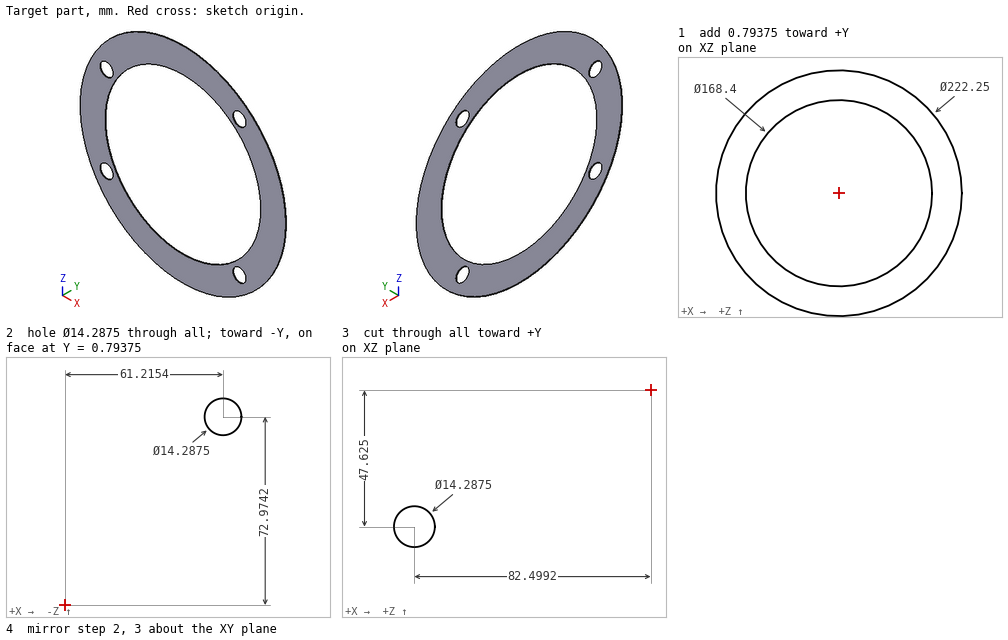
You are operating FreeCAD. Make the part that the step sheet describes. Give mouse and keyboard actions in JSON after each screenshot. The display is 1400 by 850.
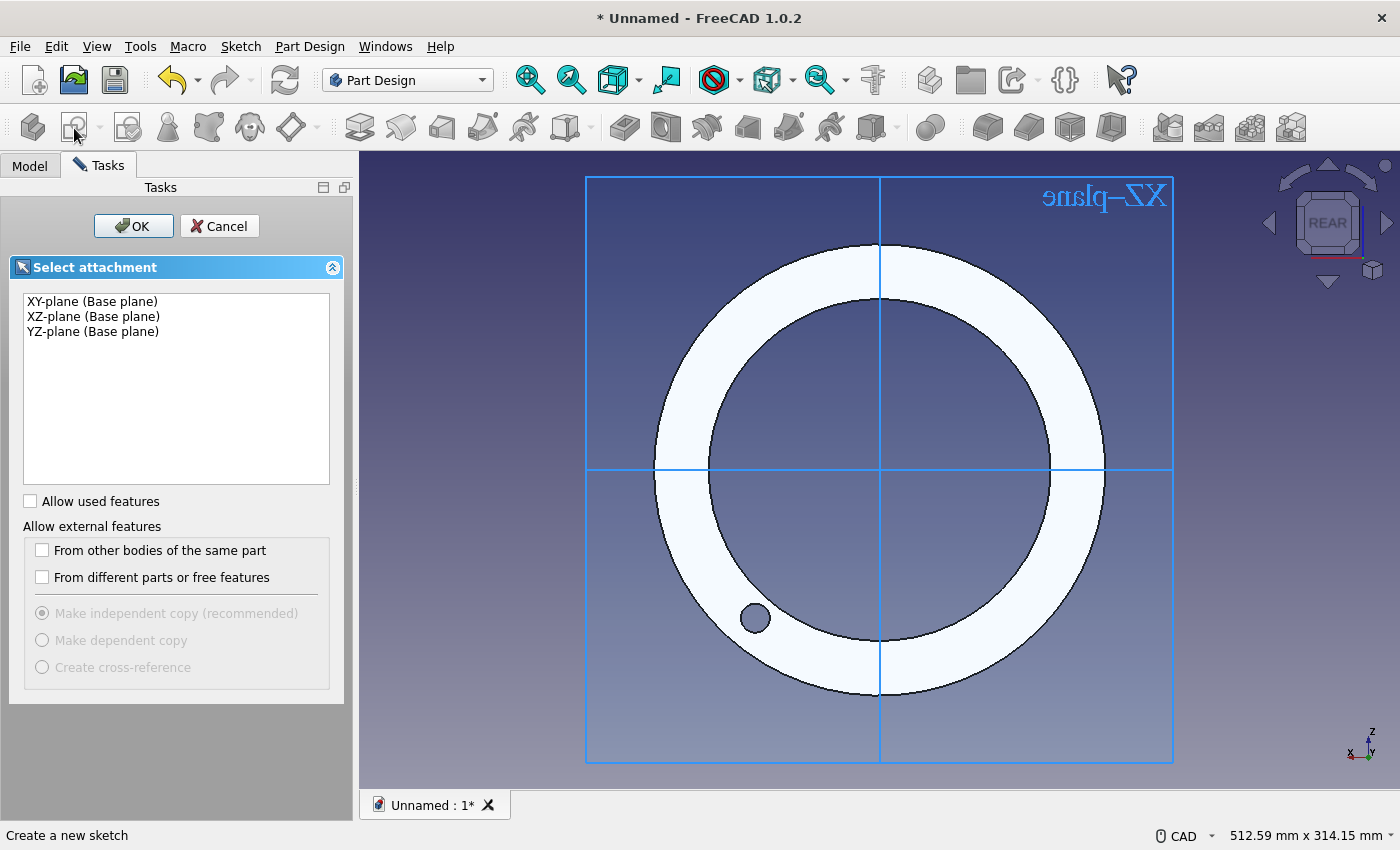
{"action": "left_click", "coordinate": [84, 316]}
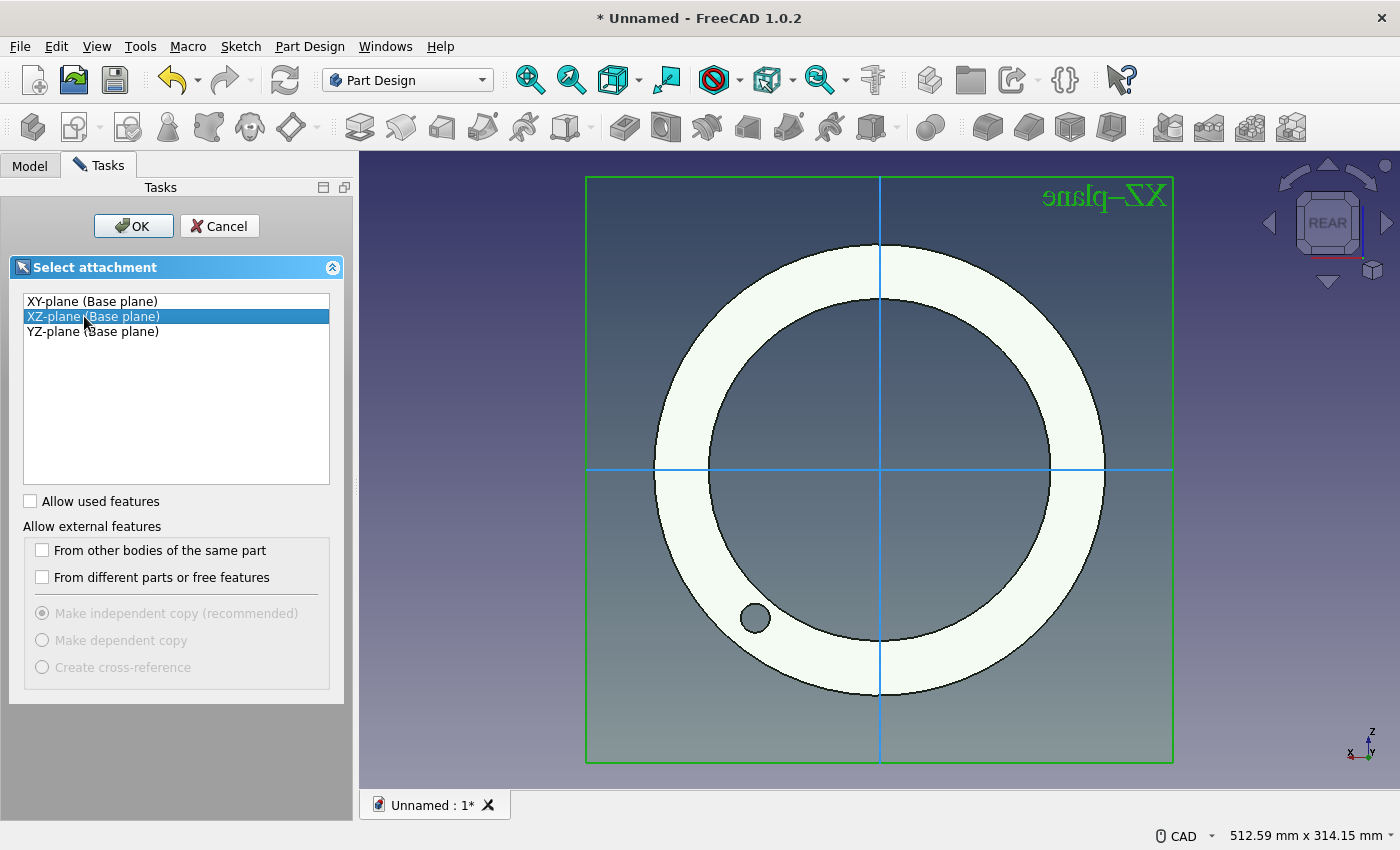
{"action": "left_click", "coordinate": [134, 226]}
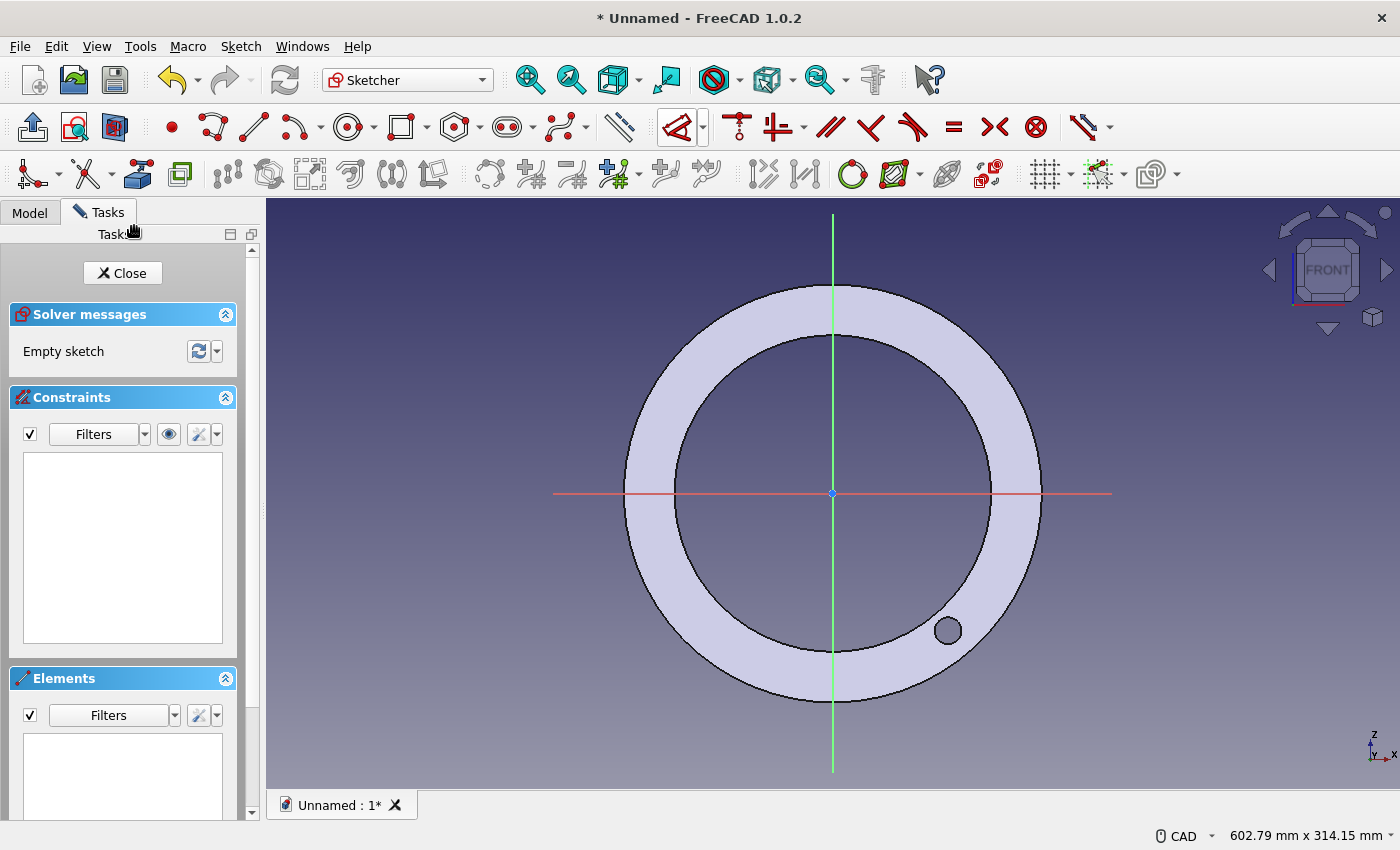
{"action": "scroll", "coordinate": [671, 590], "scroll_direction": "up", "scroll_amount": 13}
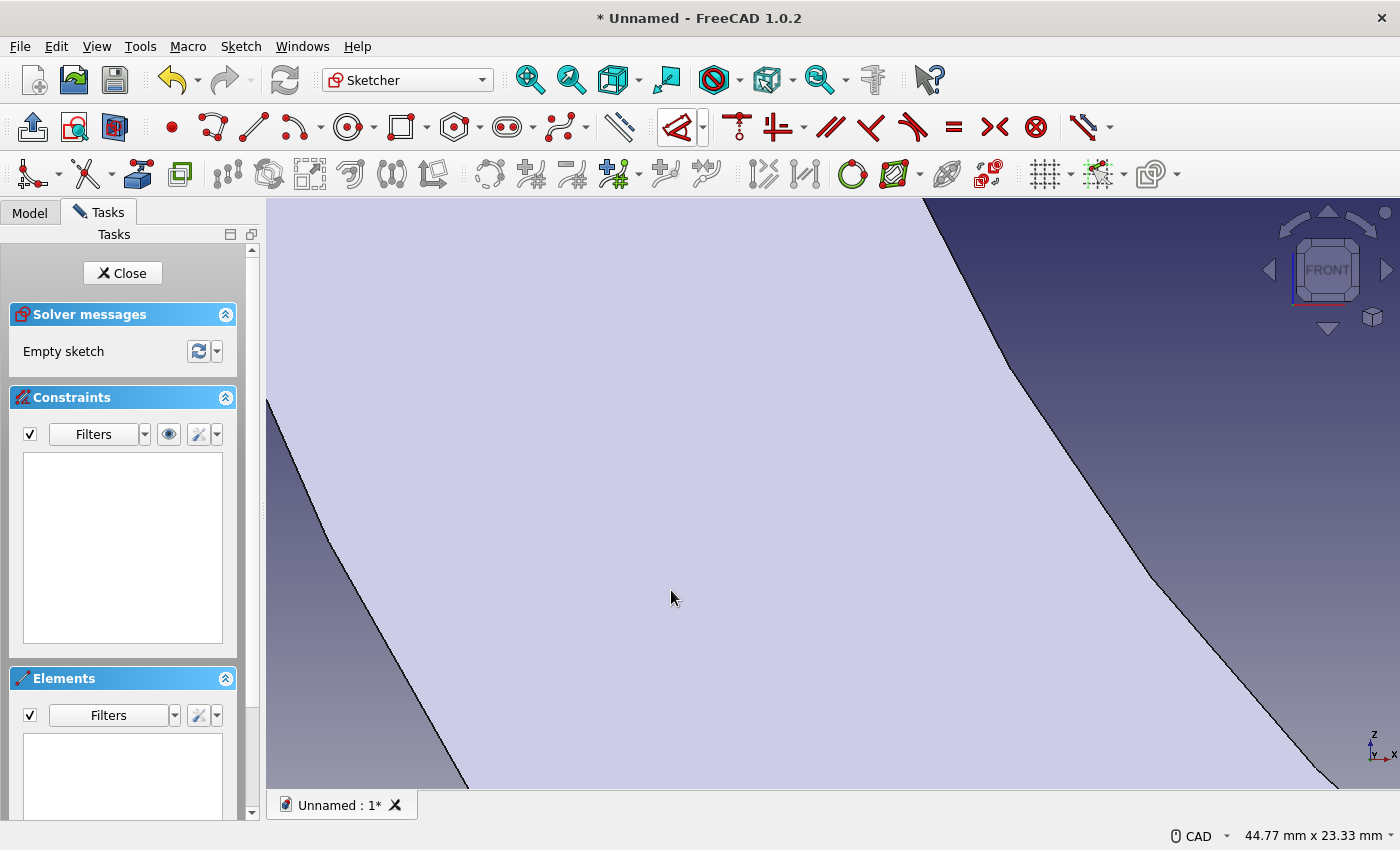
{"action": "left_click", "coordinate": [348, 128]}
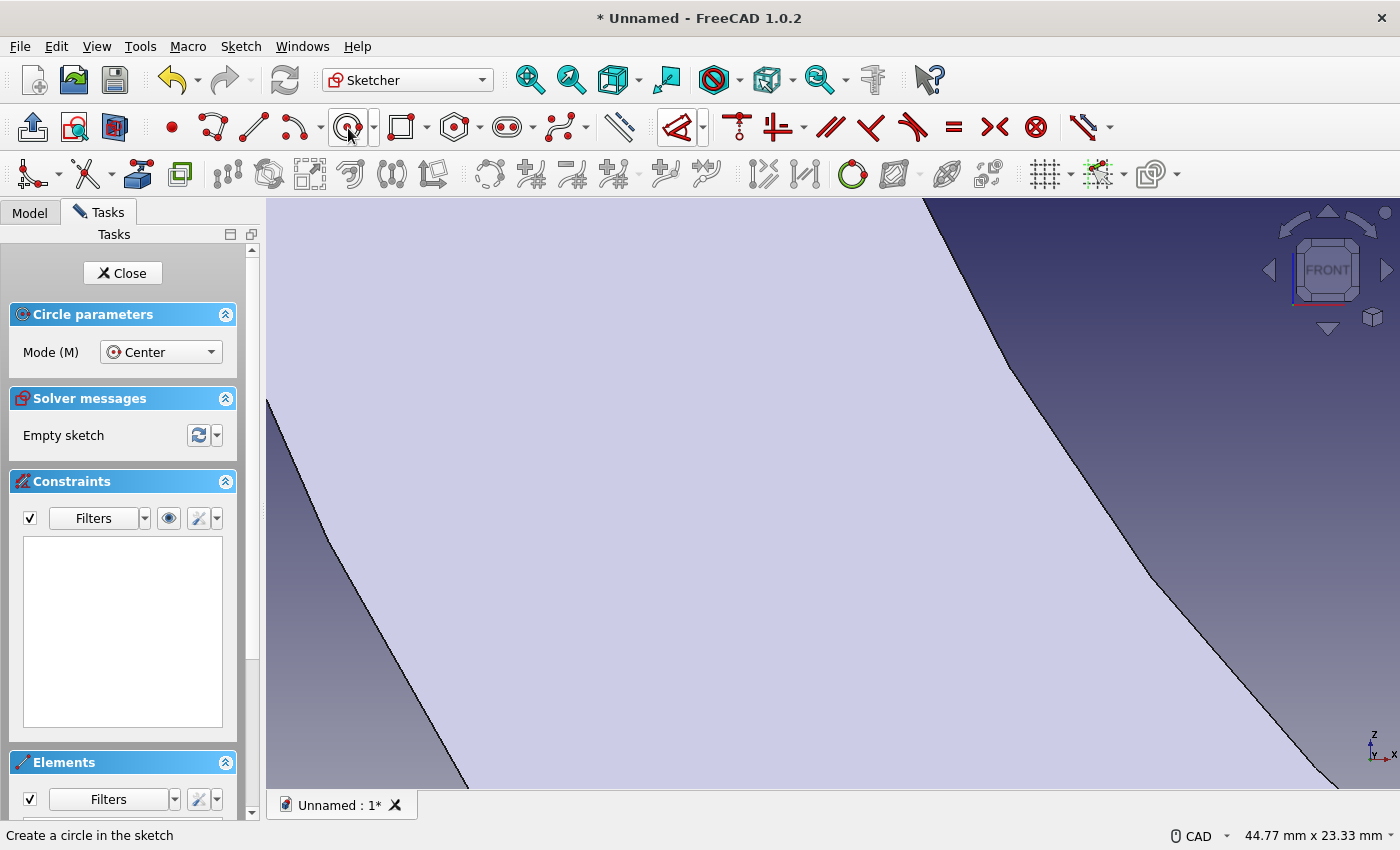
{"action": "left_click", "coordinate": [756, 489]}
{"action": "left_click", "coordinate": [884, 361]}
{"action": "key", "text": "Escape"}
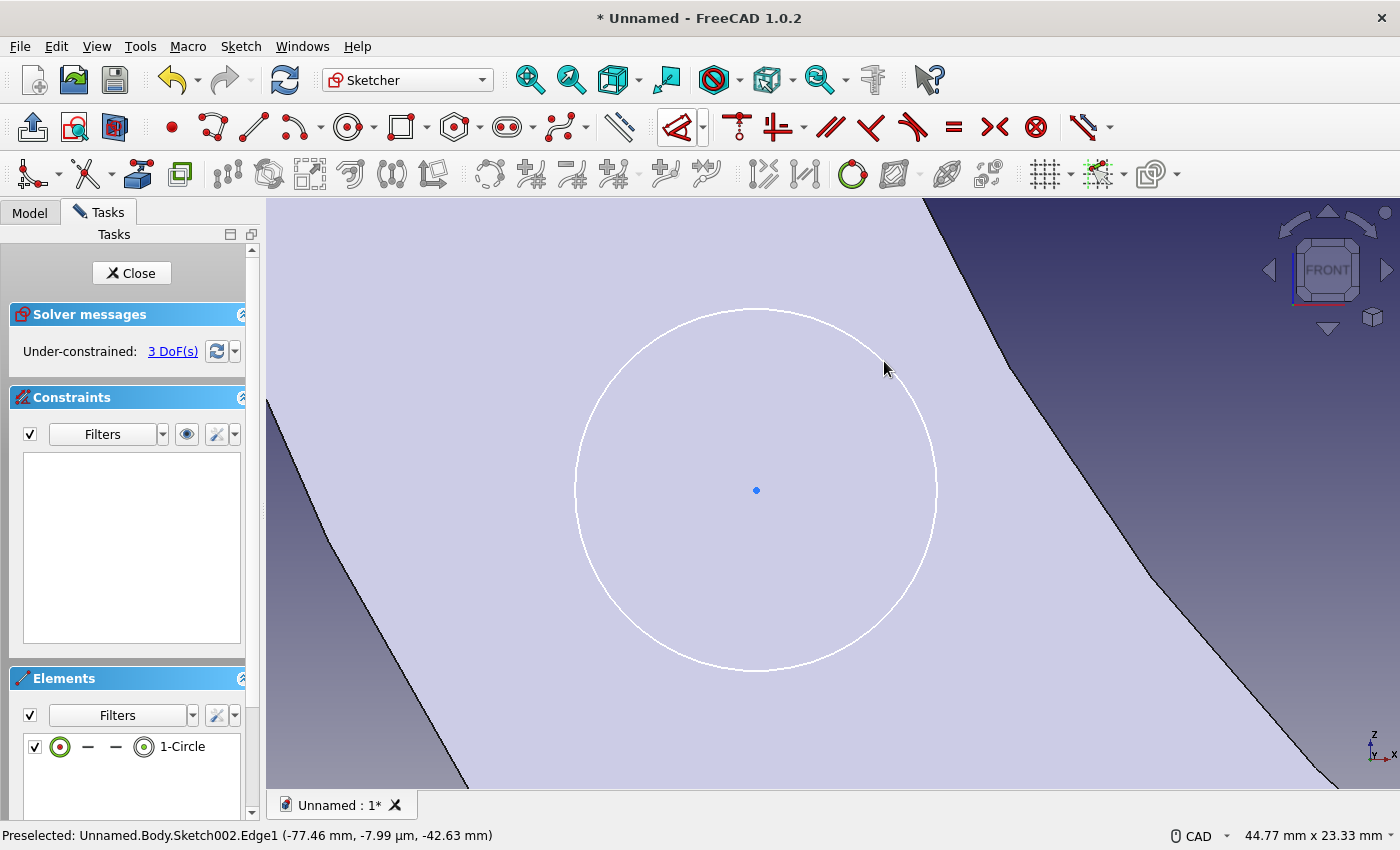
{"action": "left_click", "coordinate": [884, 362]}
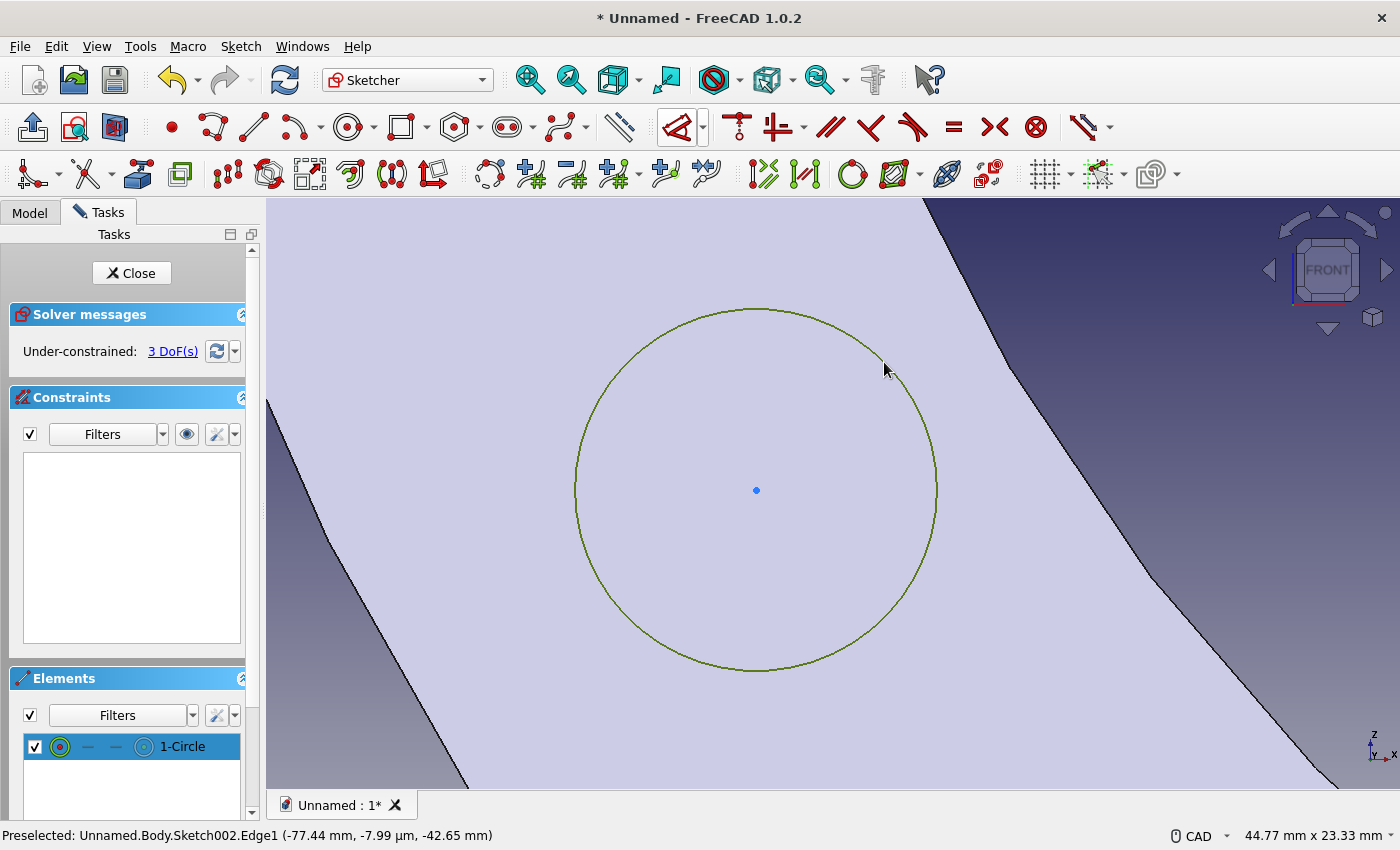
{"action": "key", "text": "k o"}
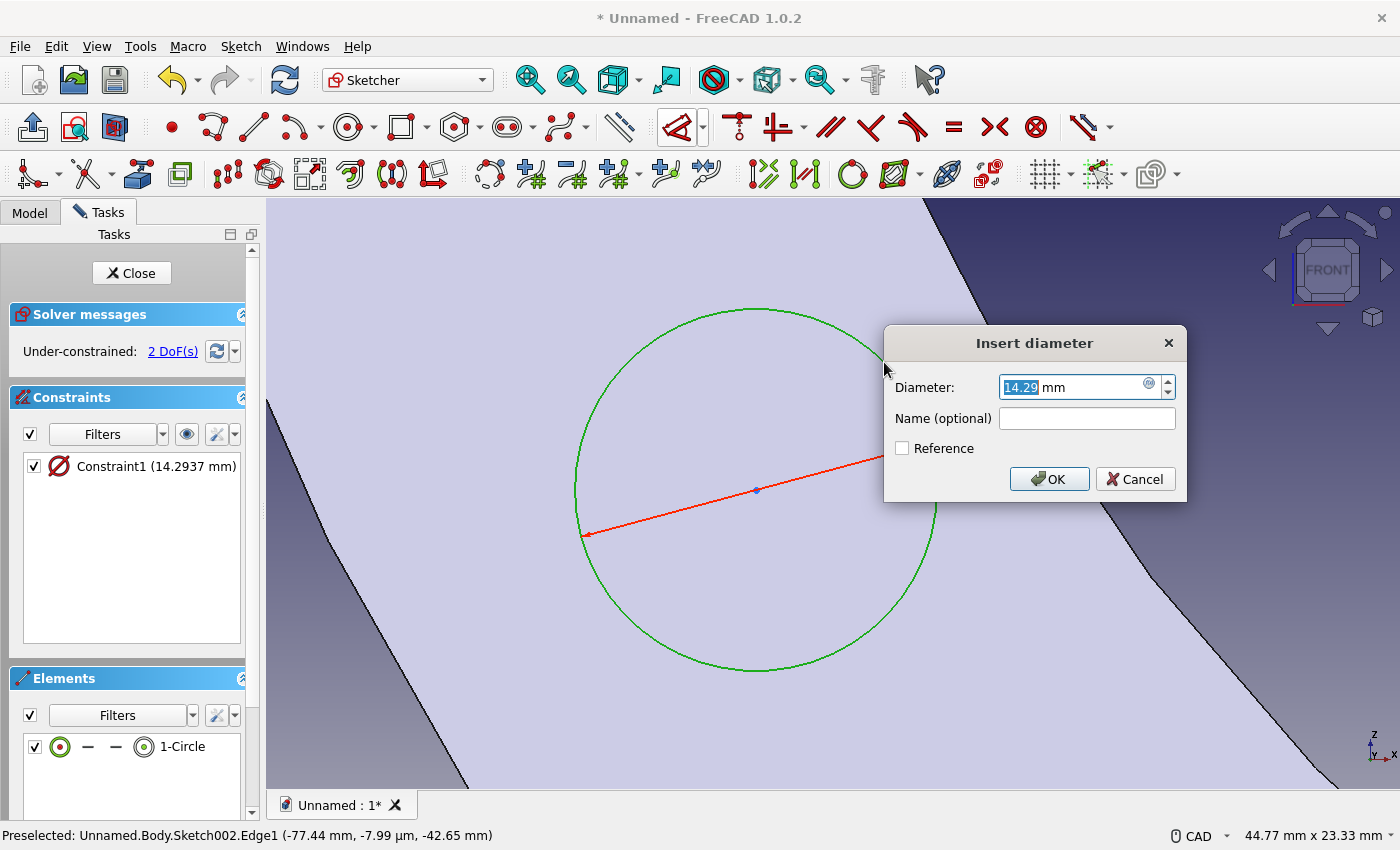
{"action": "type", "text": "14.2875"}
{"action": "key", "text": "Return"}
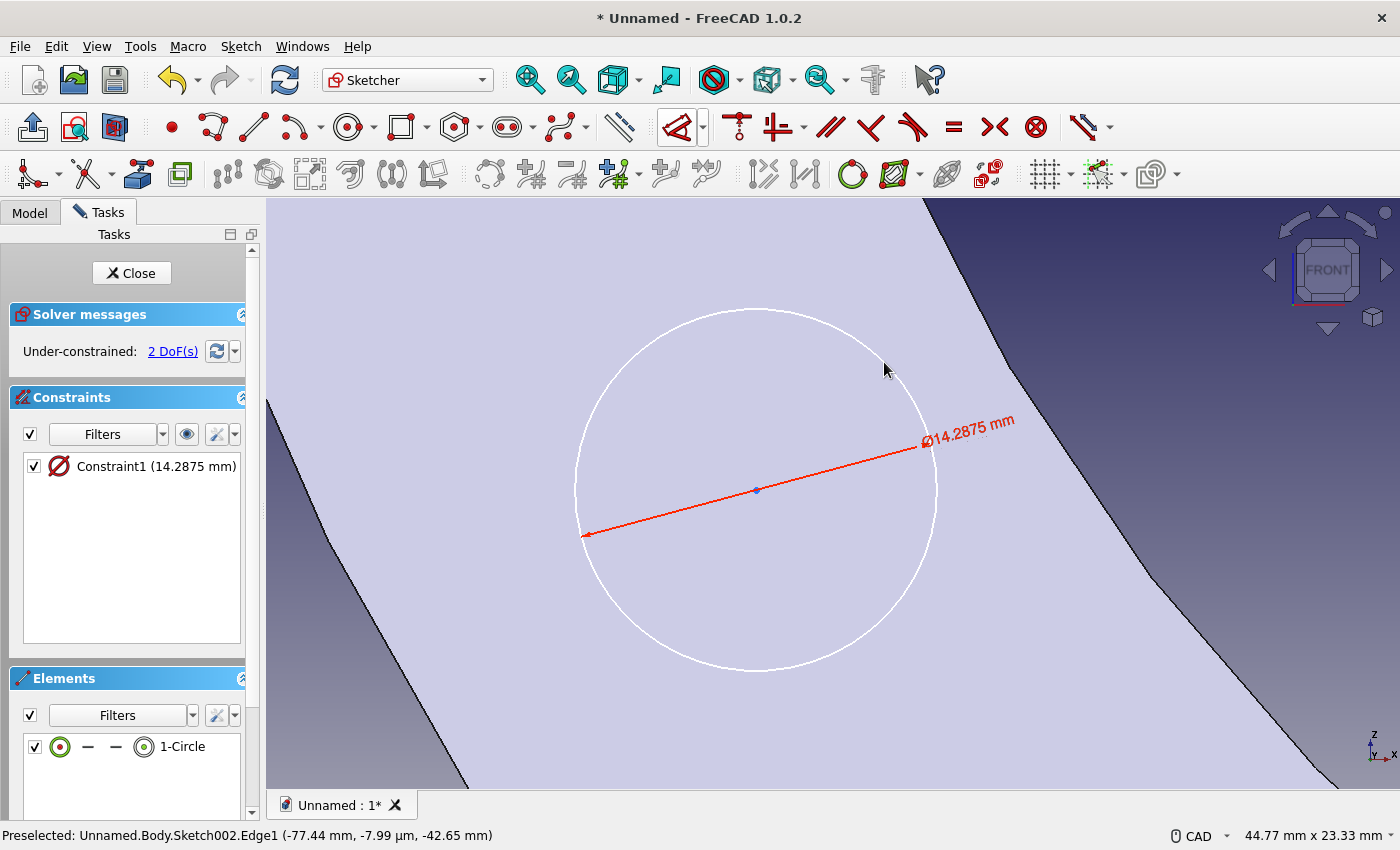
{"action": "left_click", "coordinate": [756, 490]}